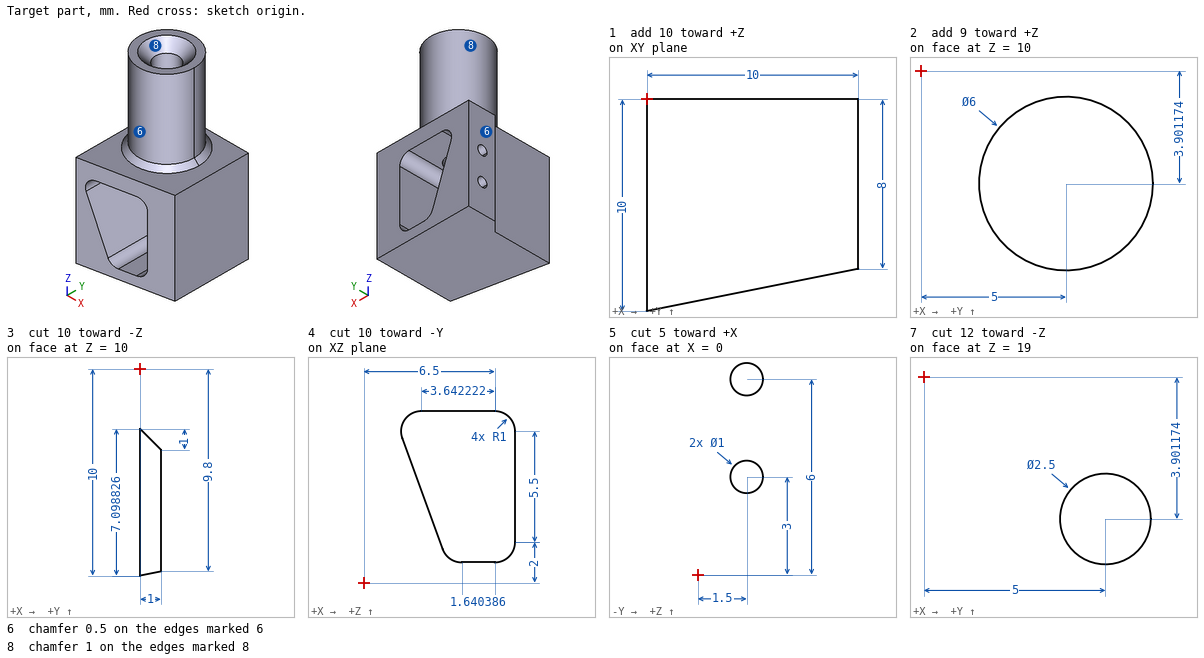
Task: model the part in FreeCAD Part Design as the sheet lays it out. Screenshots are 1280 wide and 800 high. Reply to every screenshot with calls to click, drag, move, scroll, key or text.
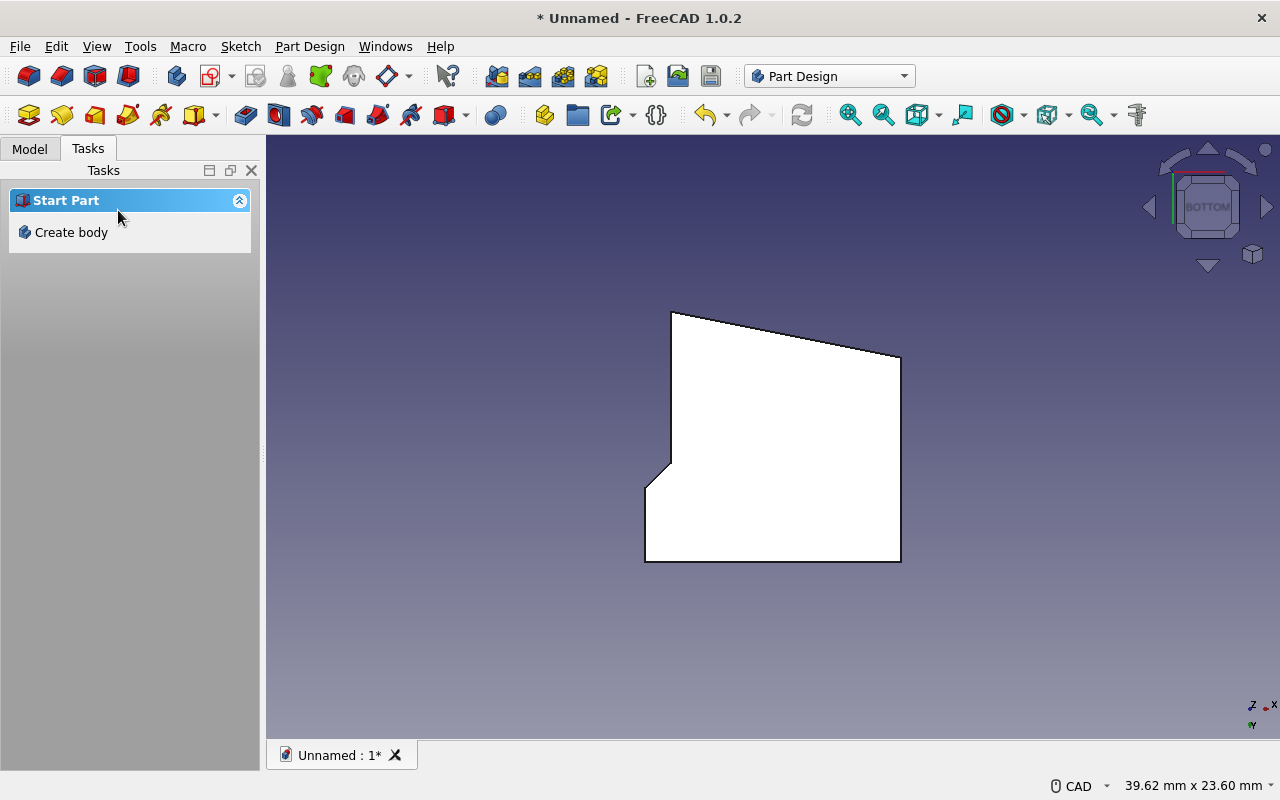
key(v)
key(f)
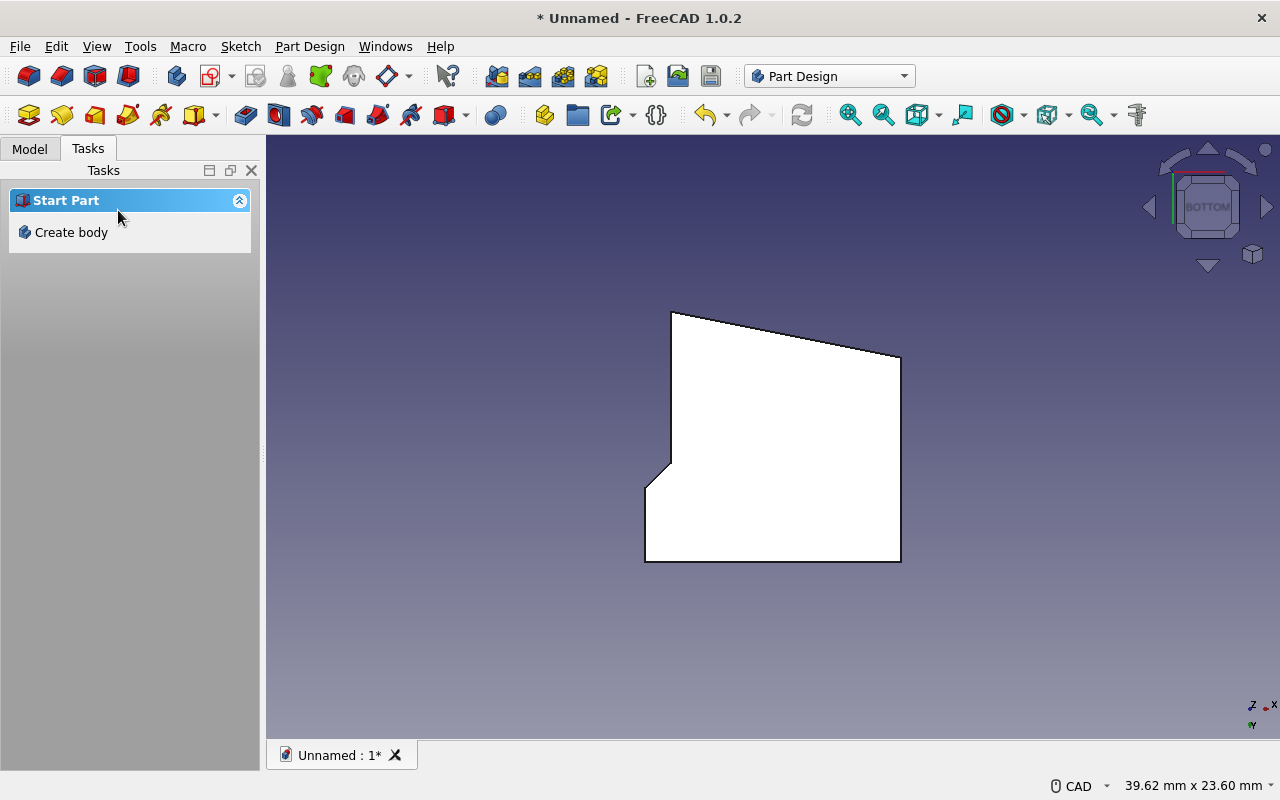
key(4)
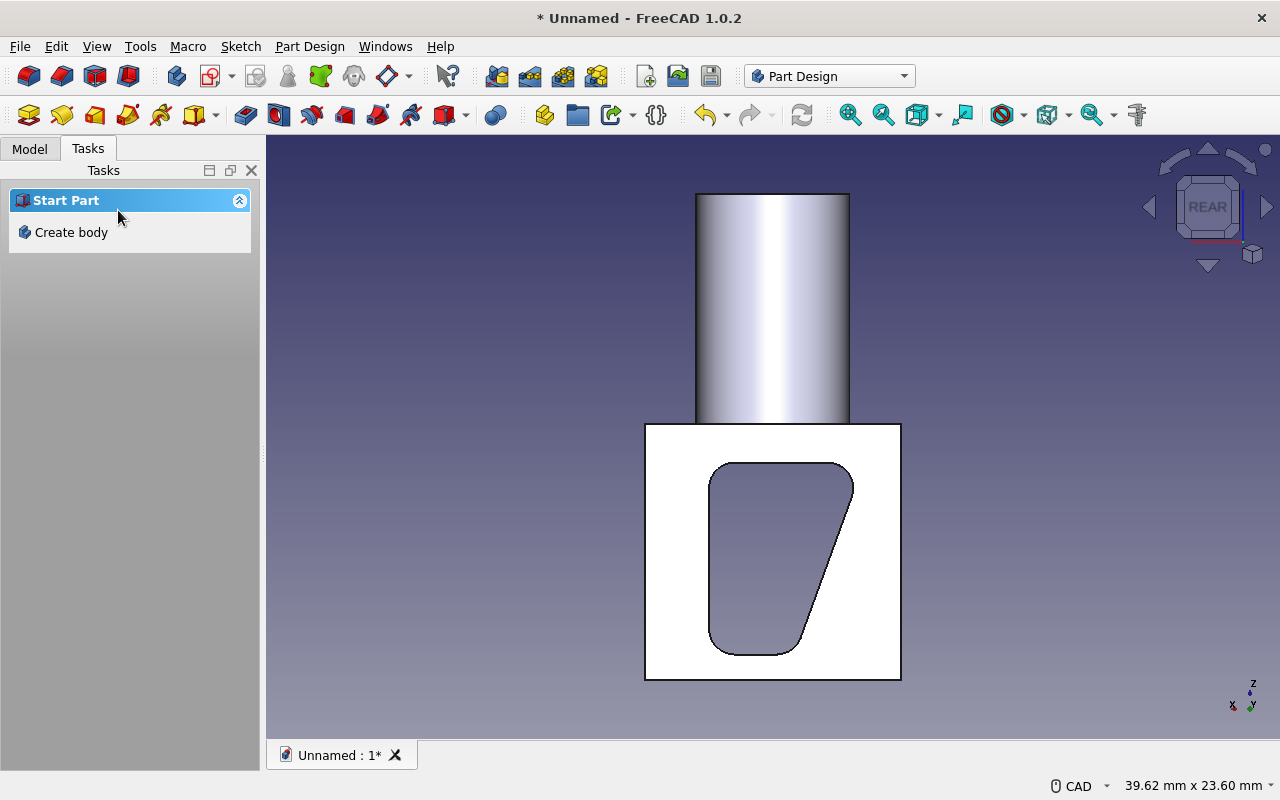
key(6)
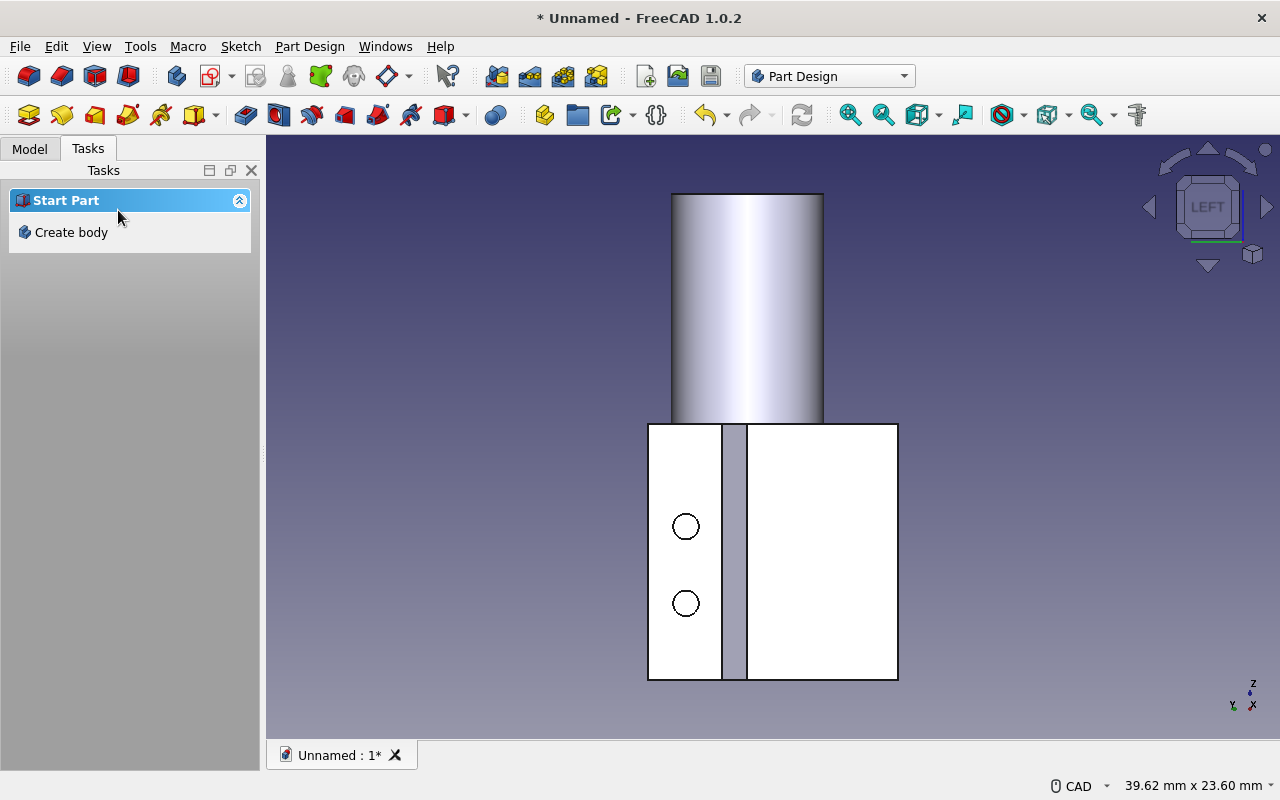
key(v)
key(3)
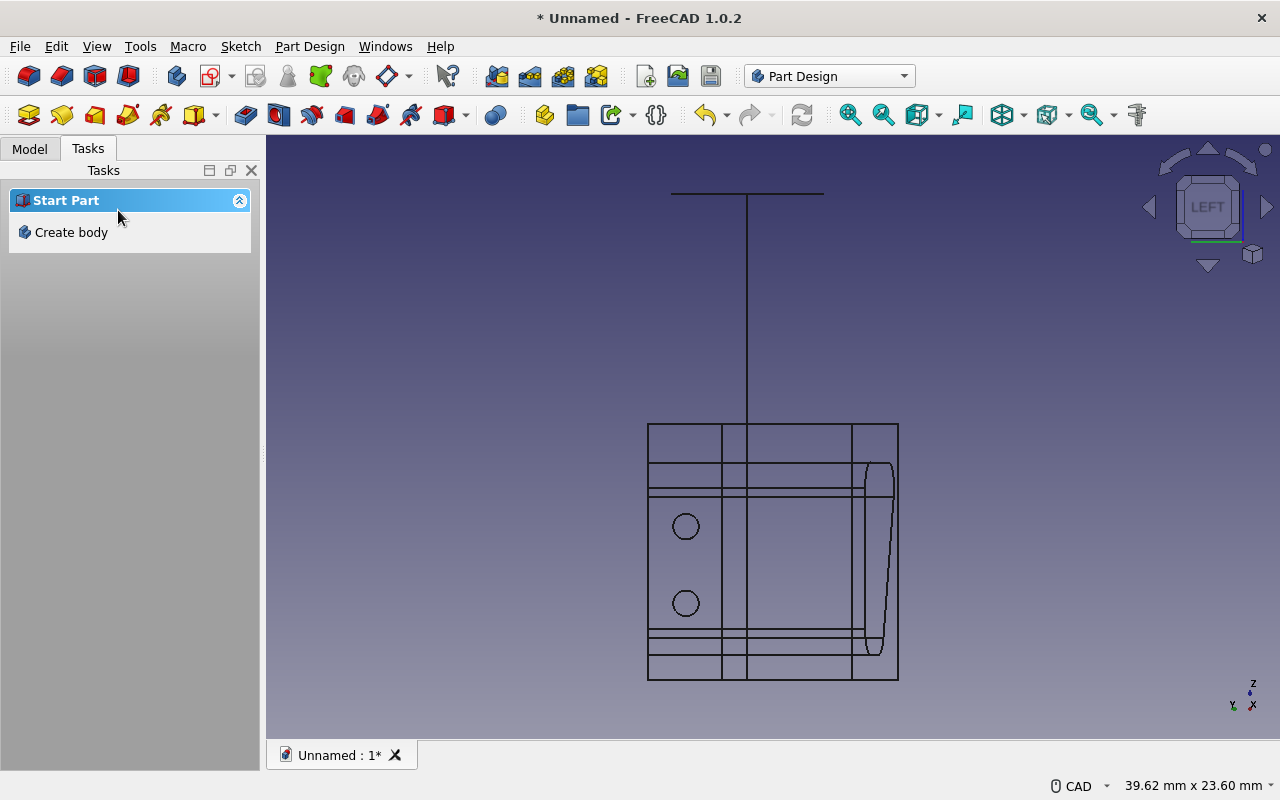
key(0)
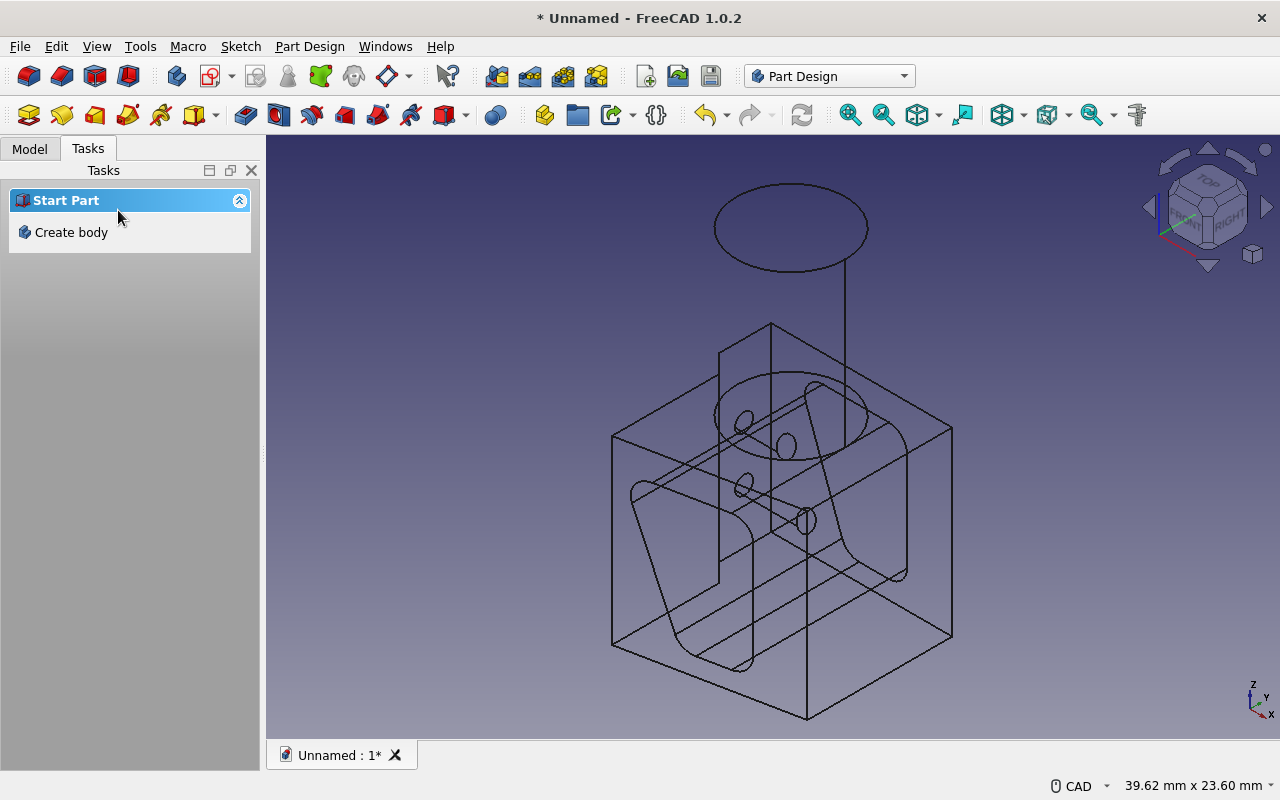
key(v)
key(f)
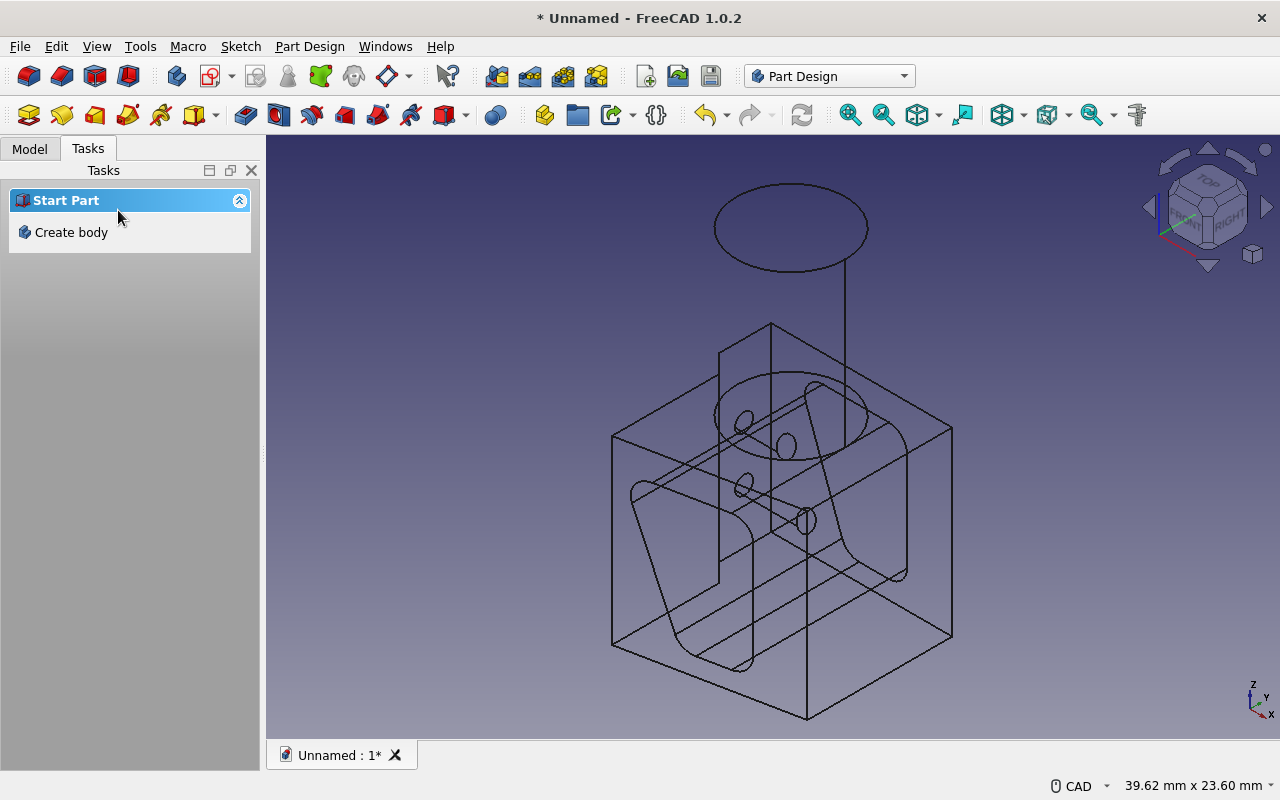
click(737, 384)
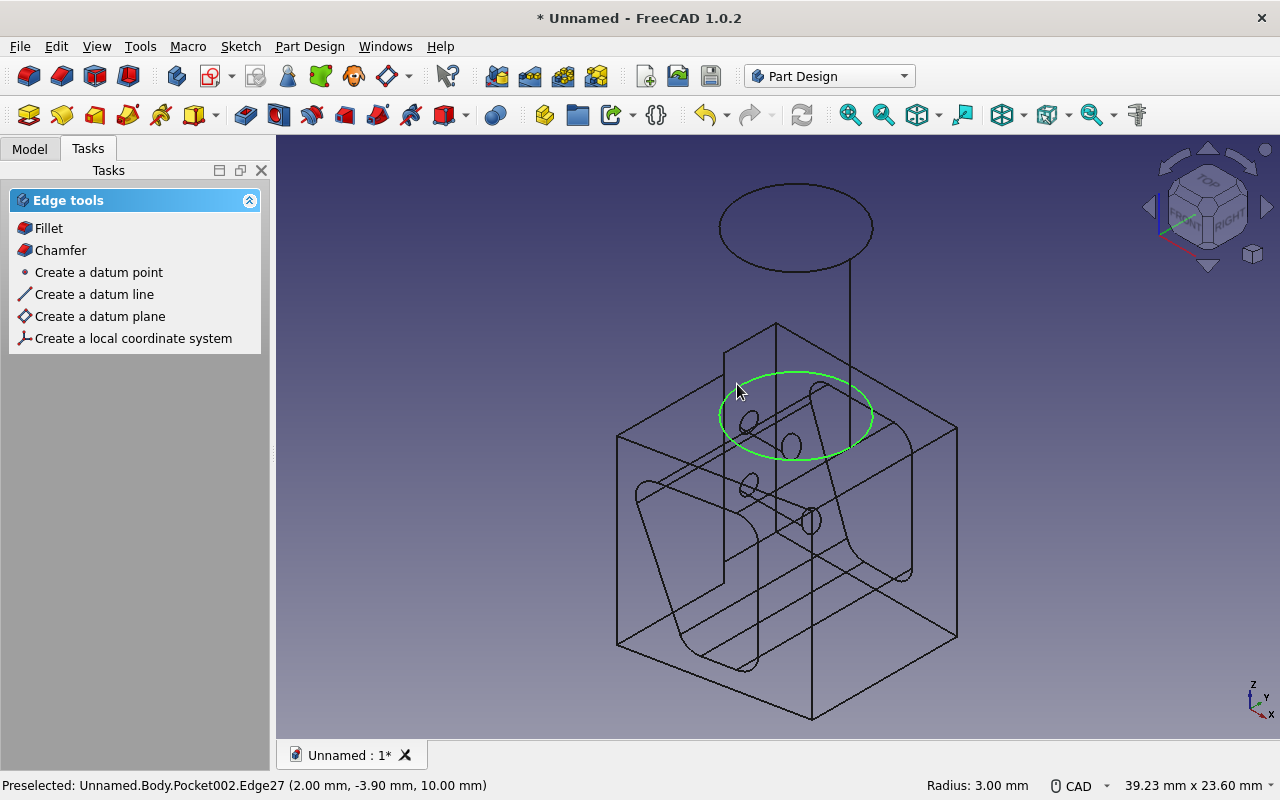
key(v)
key(1)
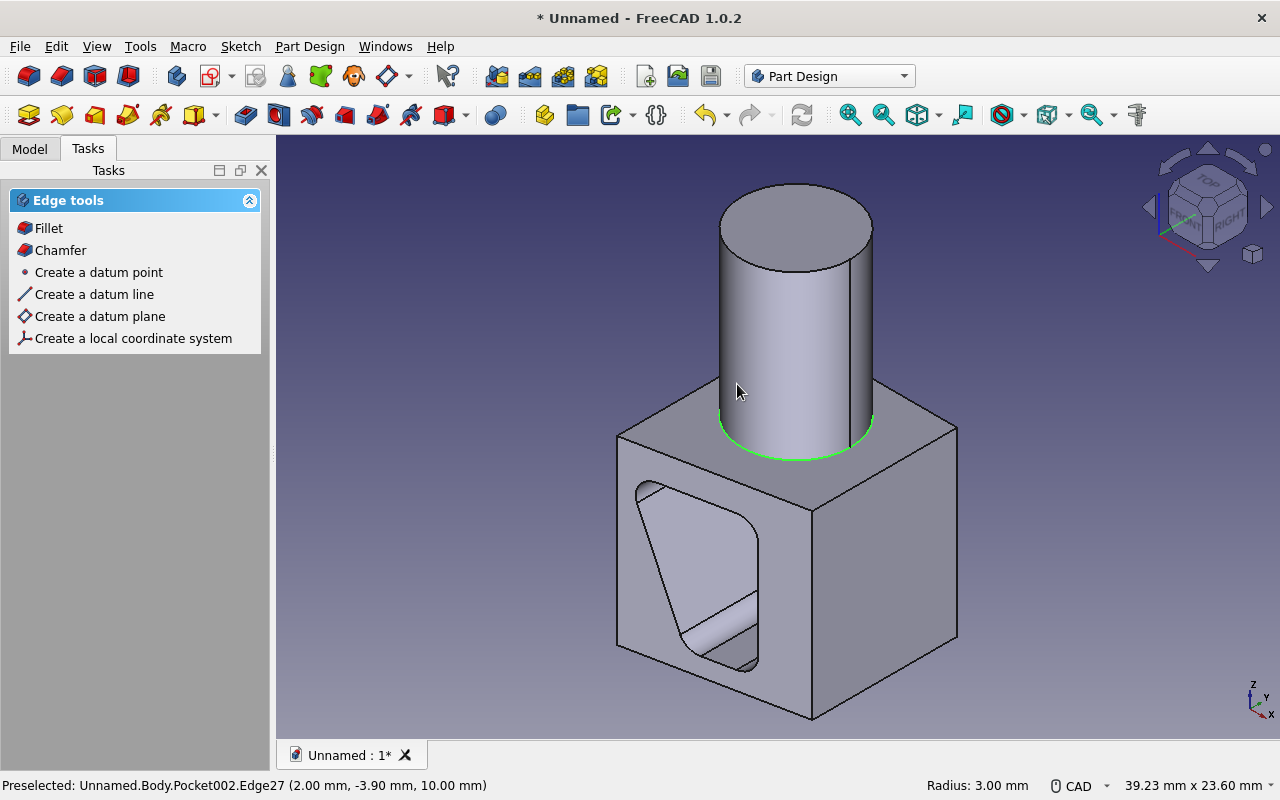
click(62, 76)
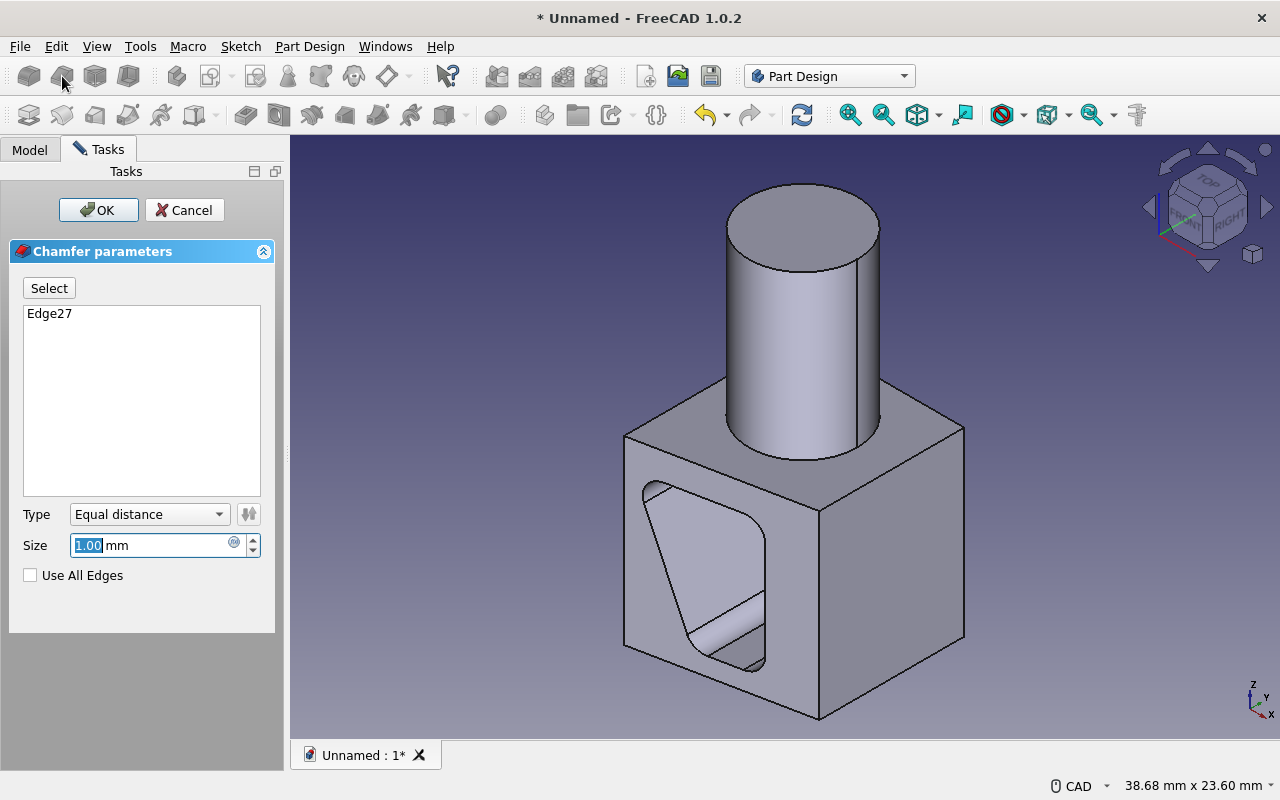
text(0.5)
key(Tab)